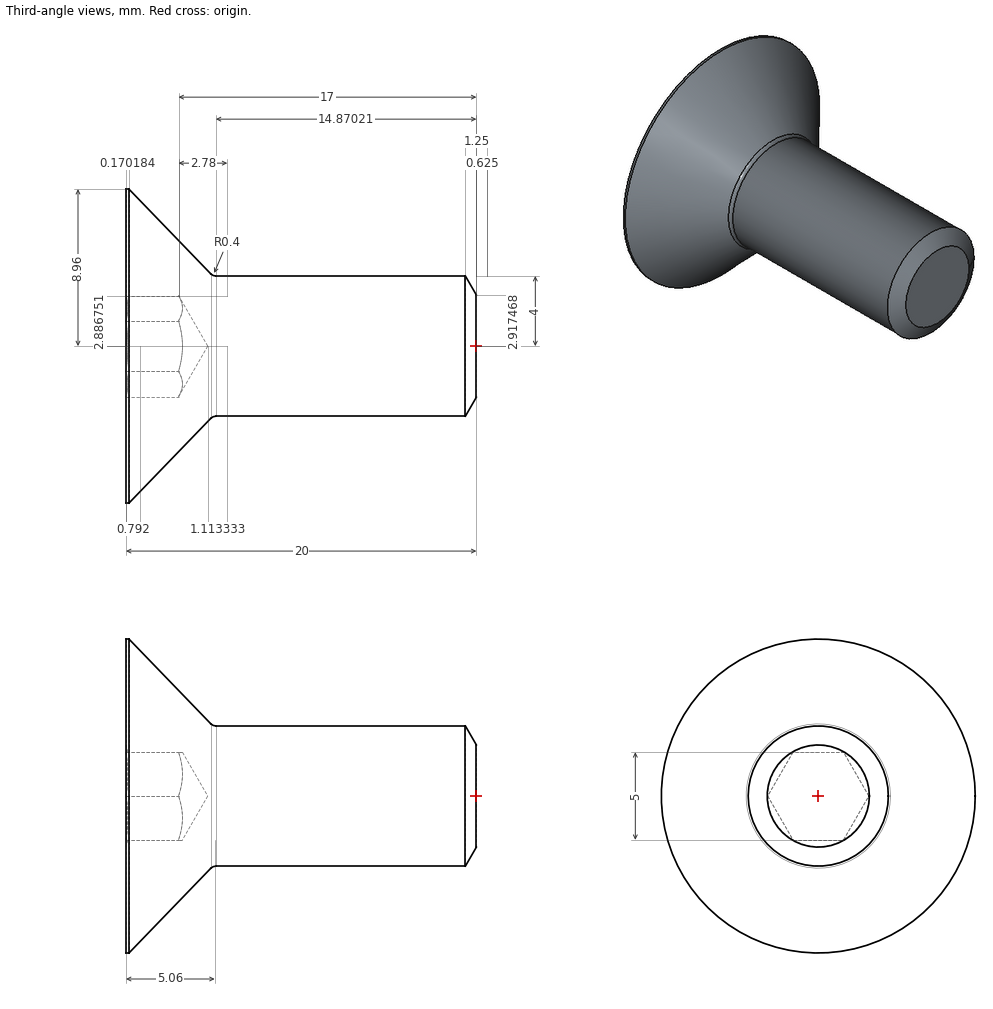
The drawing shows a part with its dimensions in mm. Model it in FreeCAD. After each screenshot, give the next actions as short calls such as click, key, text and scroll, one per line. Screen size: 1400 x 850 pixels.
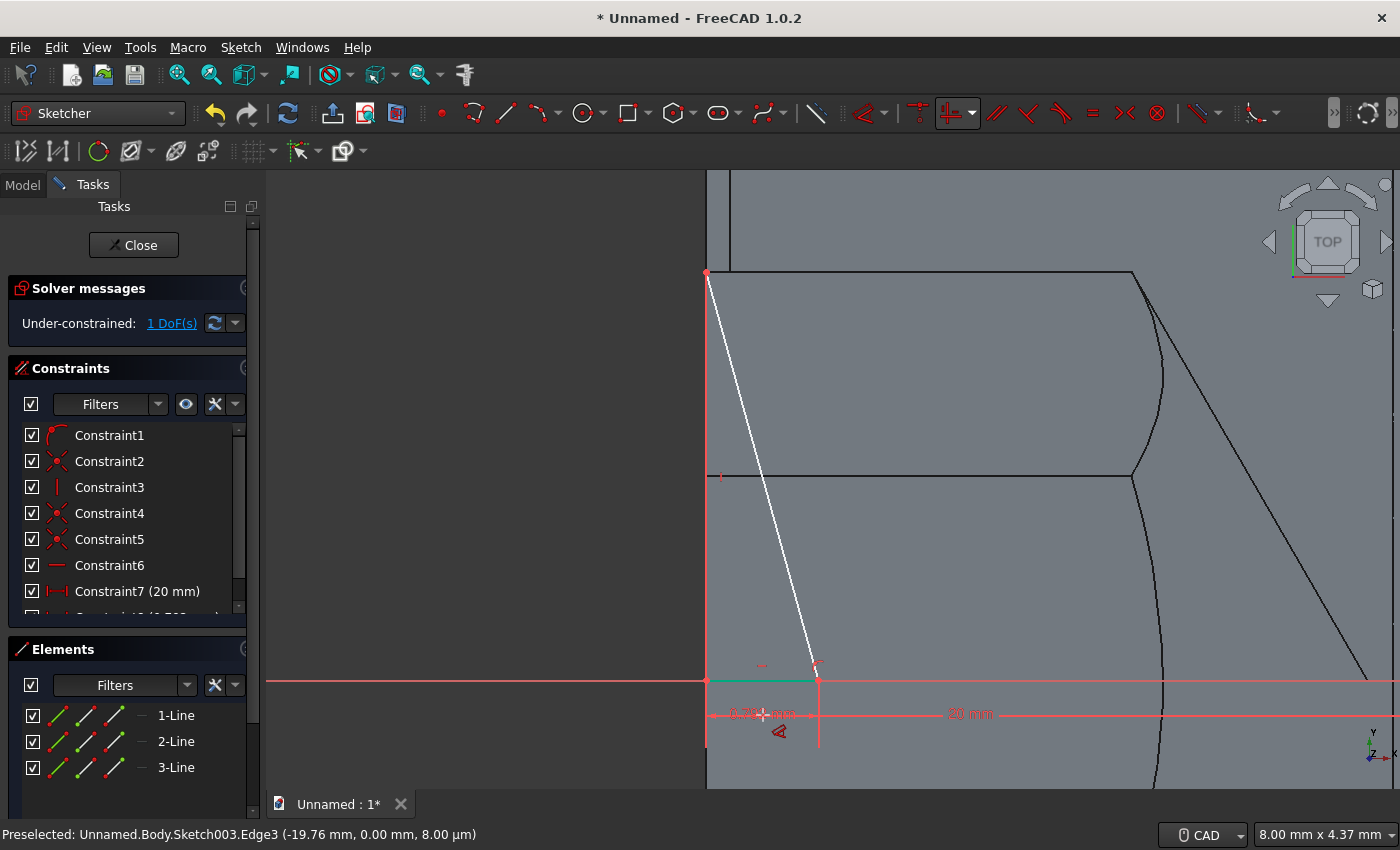
click(706, 395)
click(672, 477)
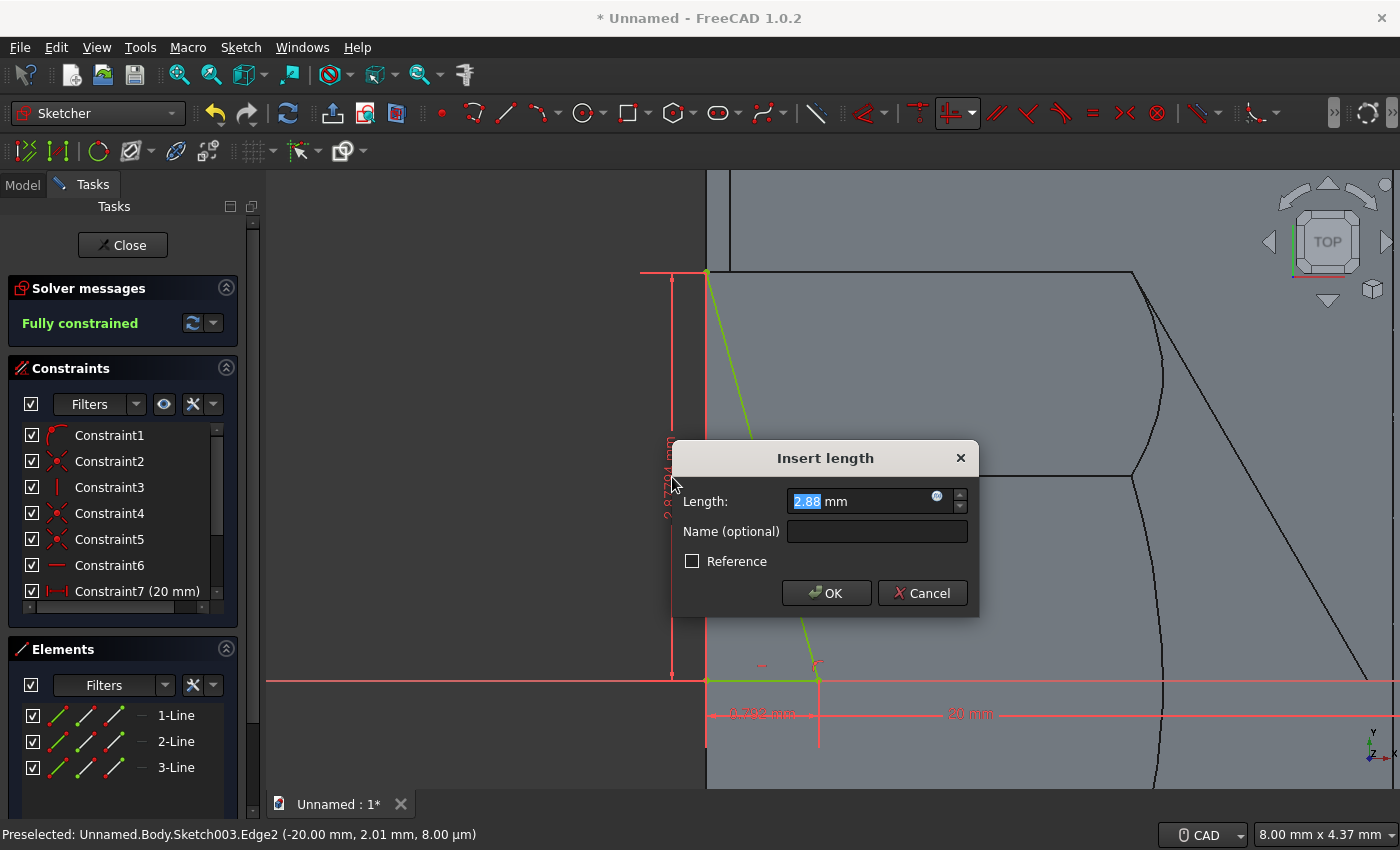
text(2.886751)
key(Return)
key(Escape)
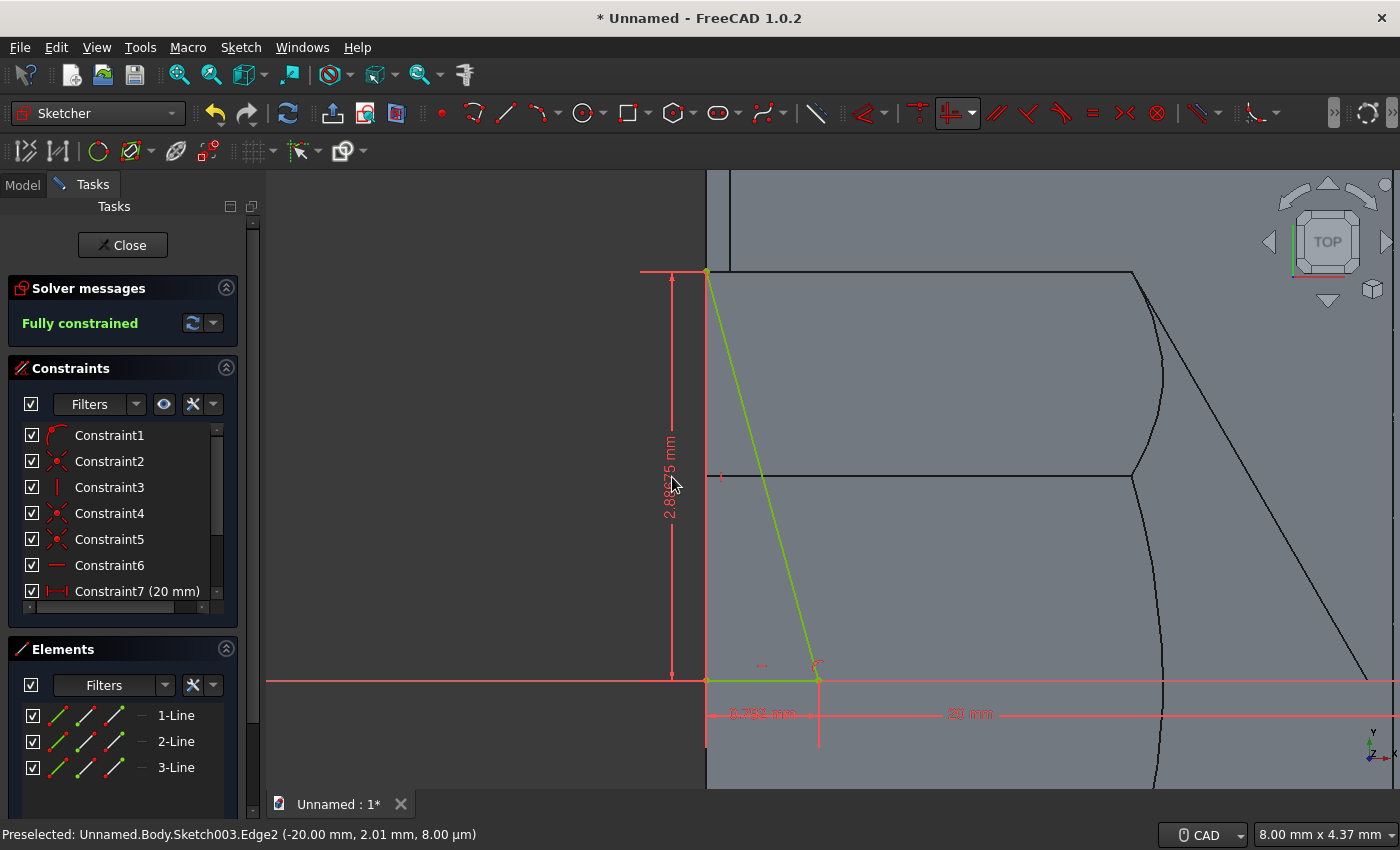
click(123, 245)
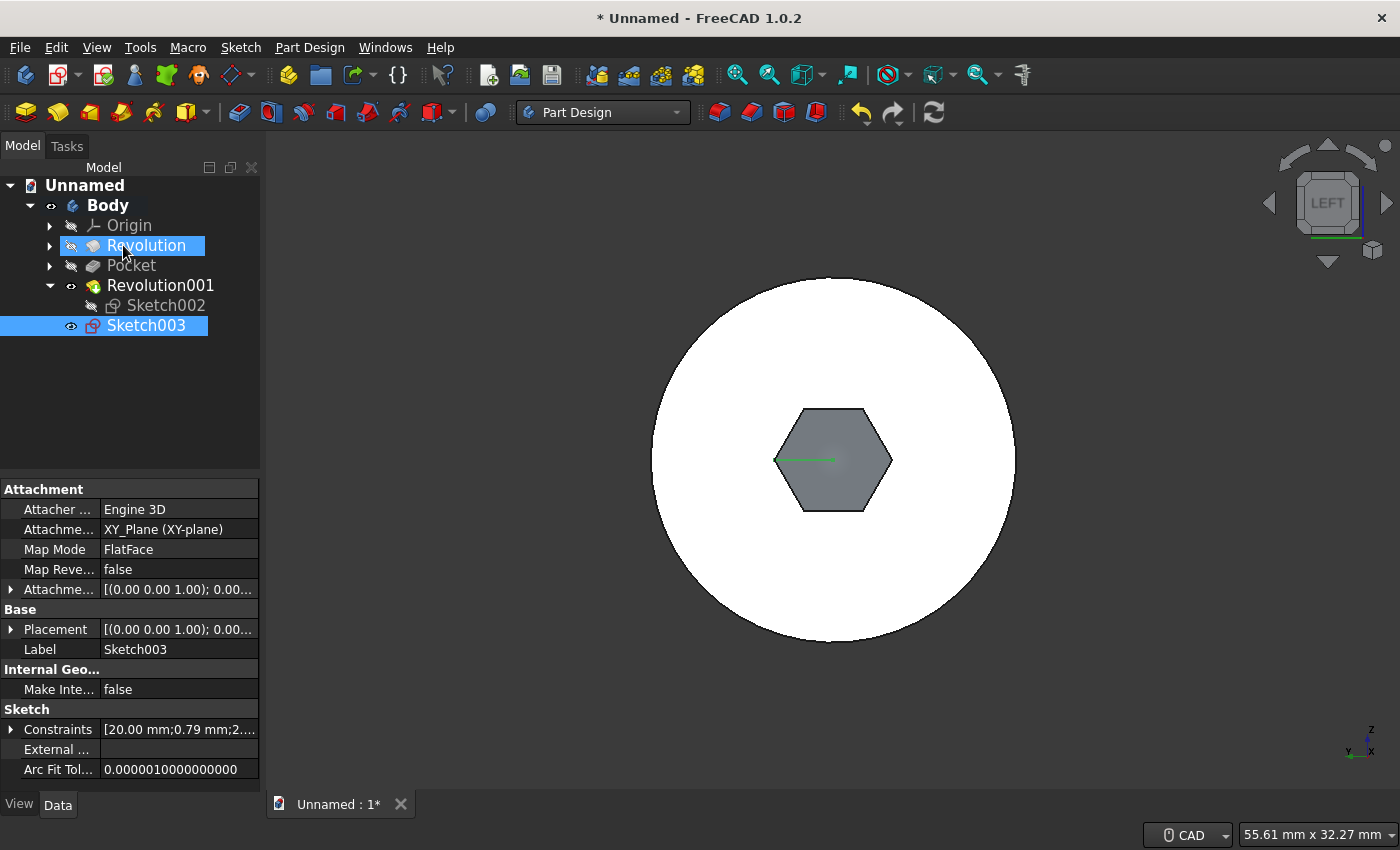
click(304, 112)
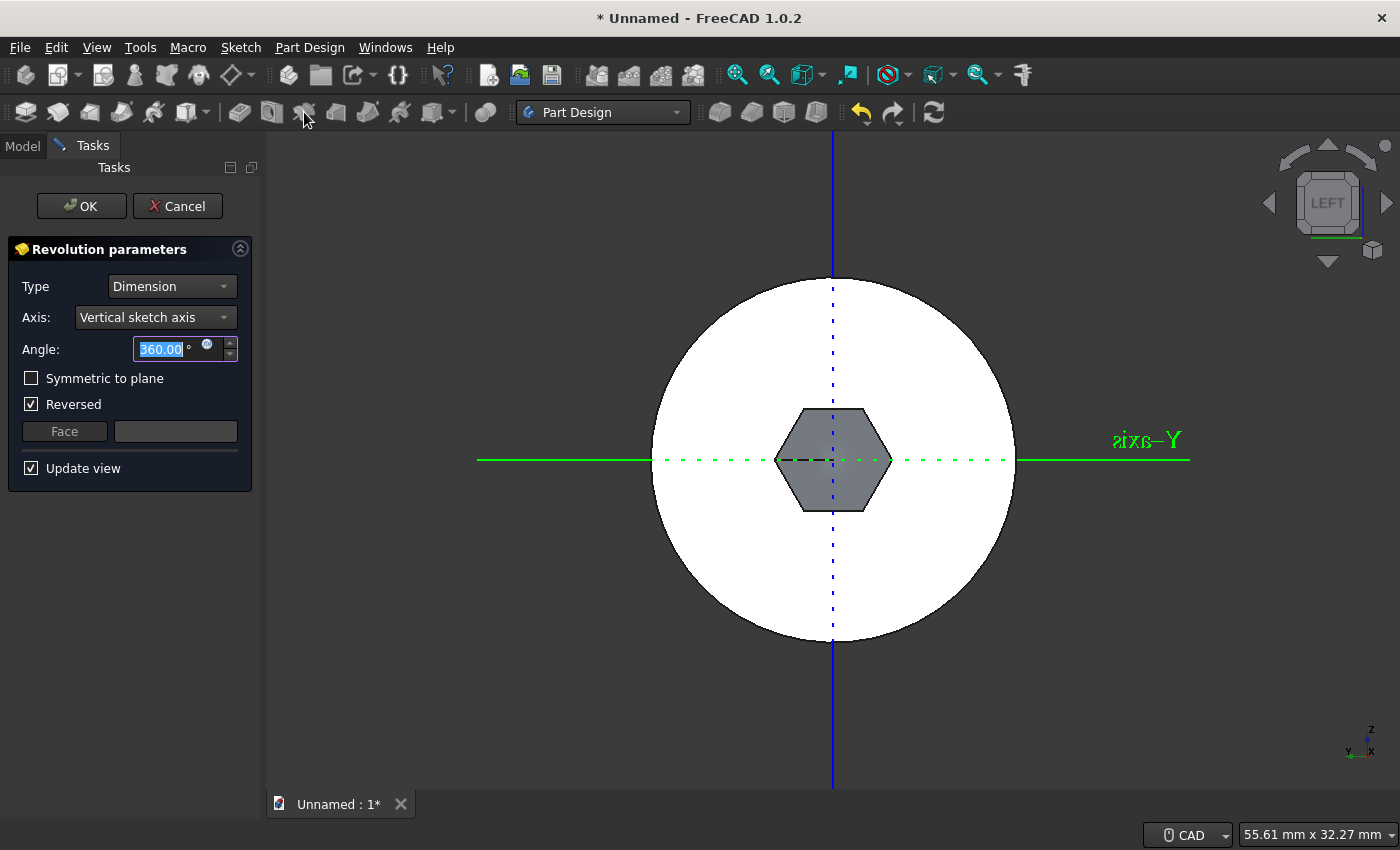
click(156, 318)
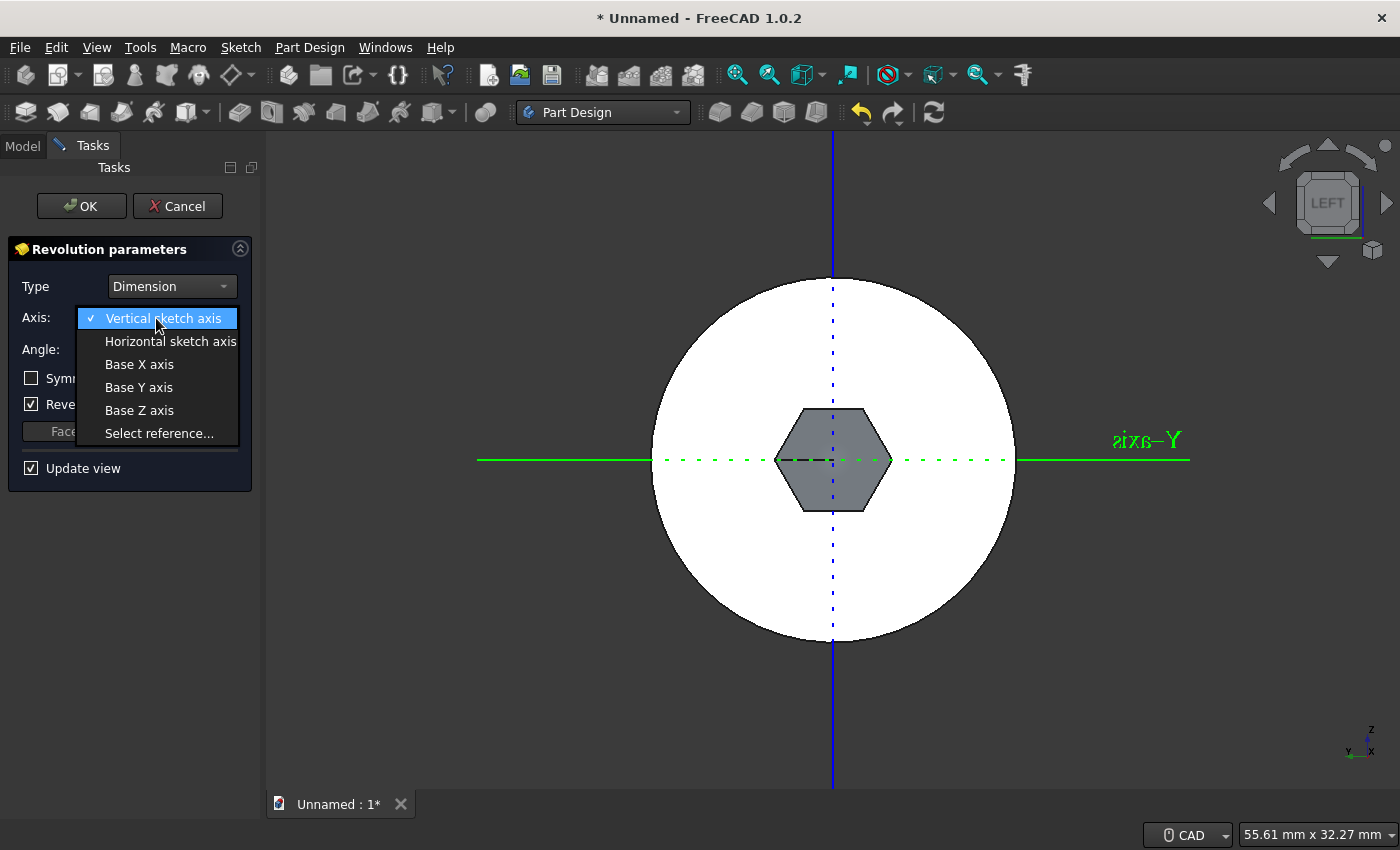
click(156, 342)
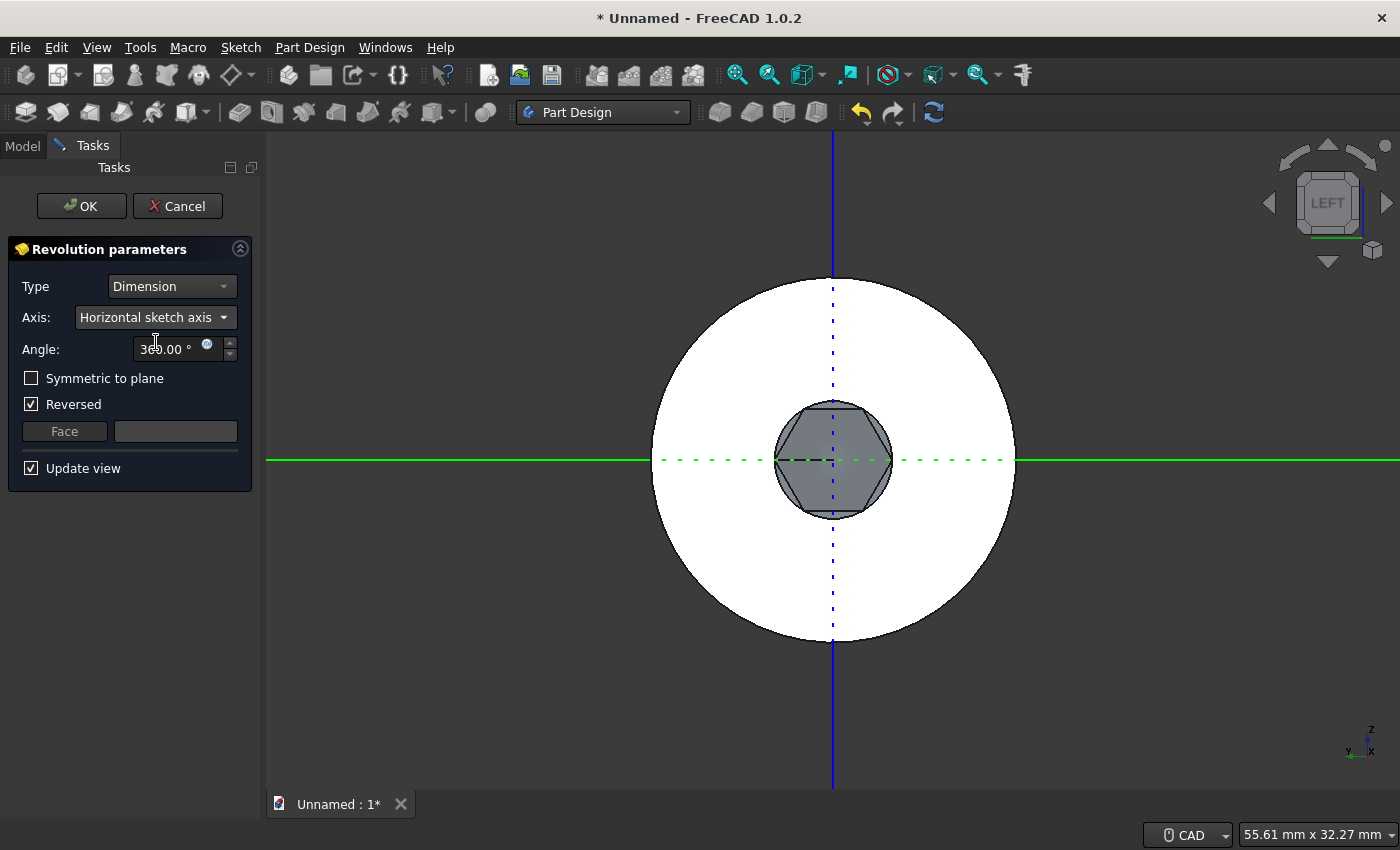
click(82, 206)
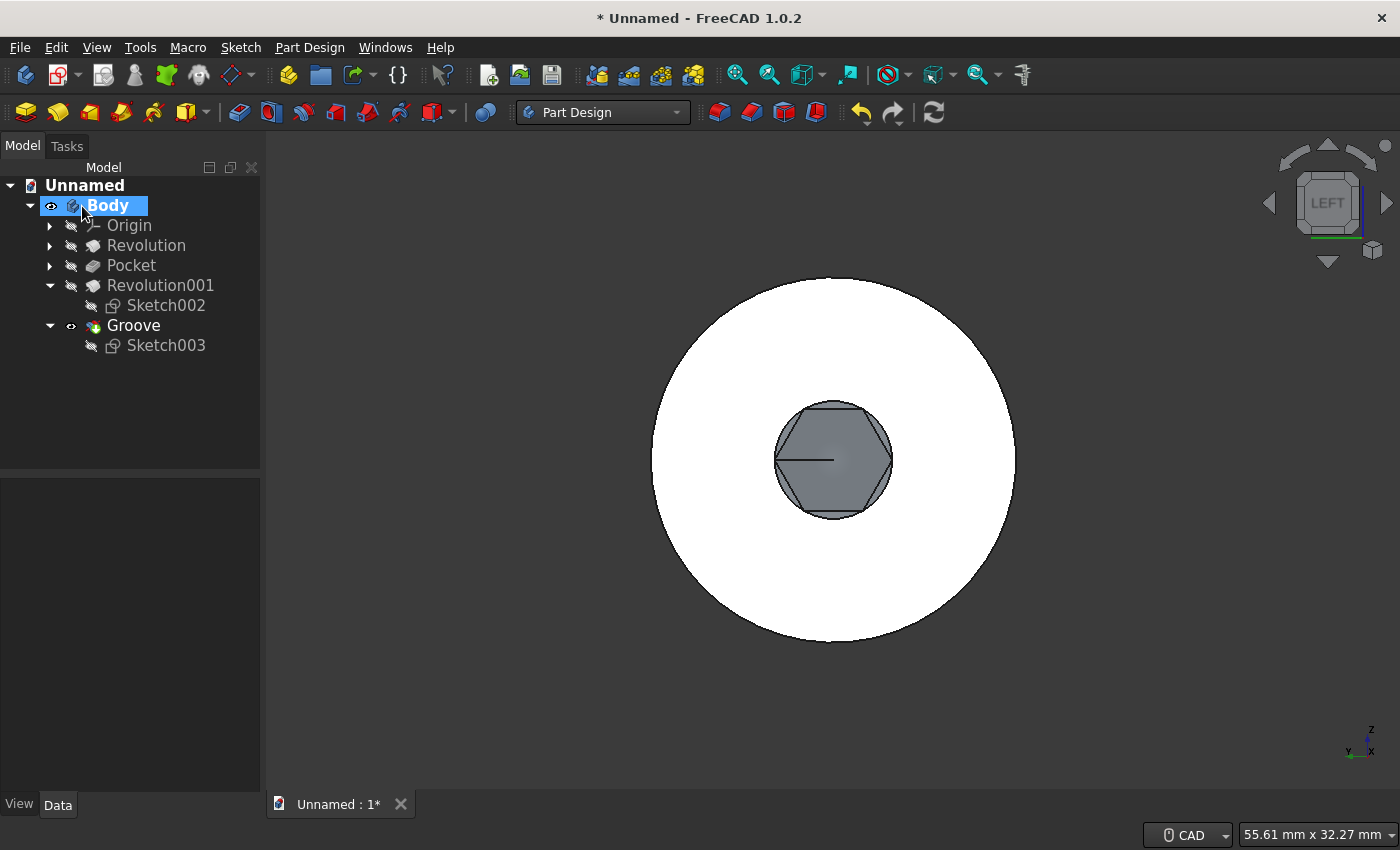
click(58, 76)